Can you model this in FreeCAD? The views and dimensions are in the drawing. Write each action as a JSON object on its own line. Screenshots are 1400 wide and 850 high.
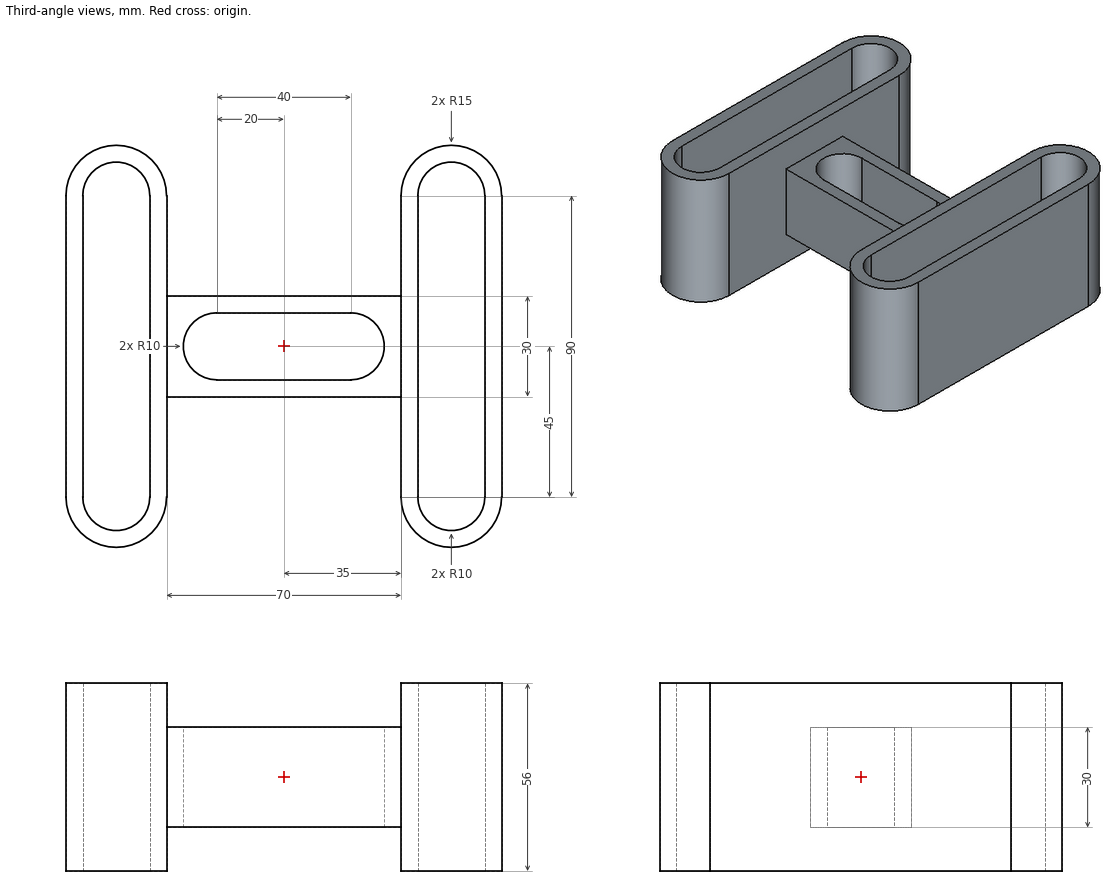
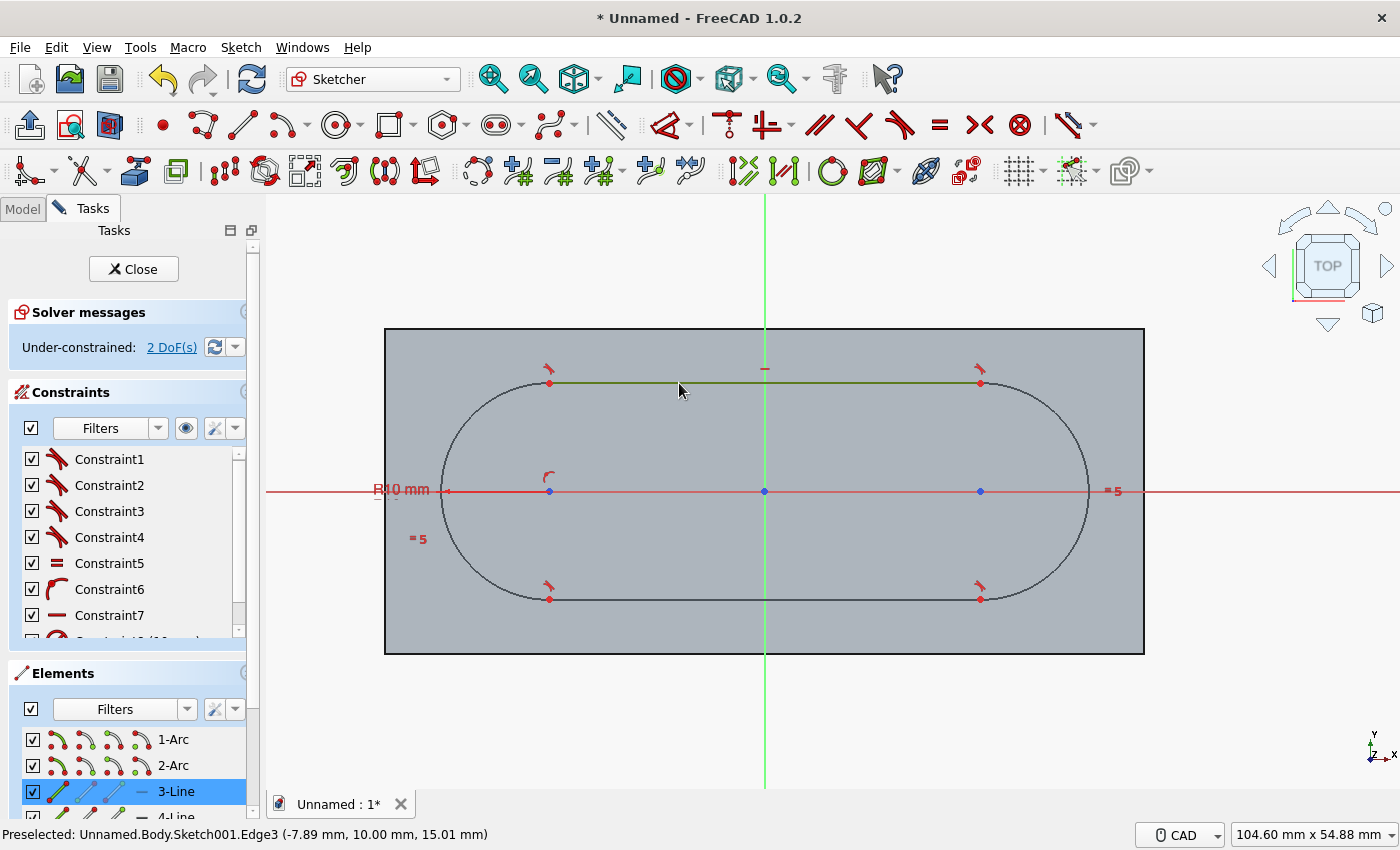
{"action": "key", "text": "l"}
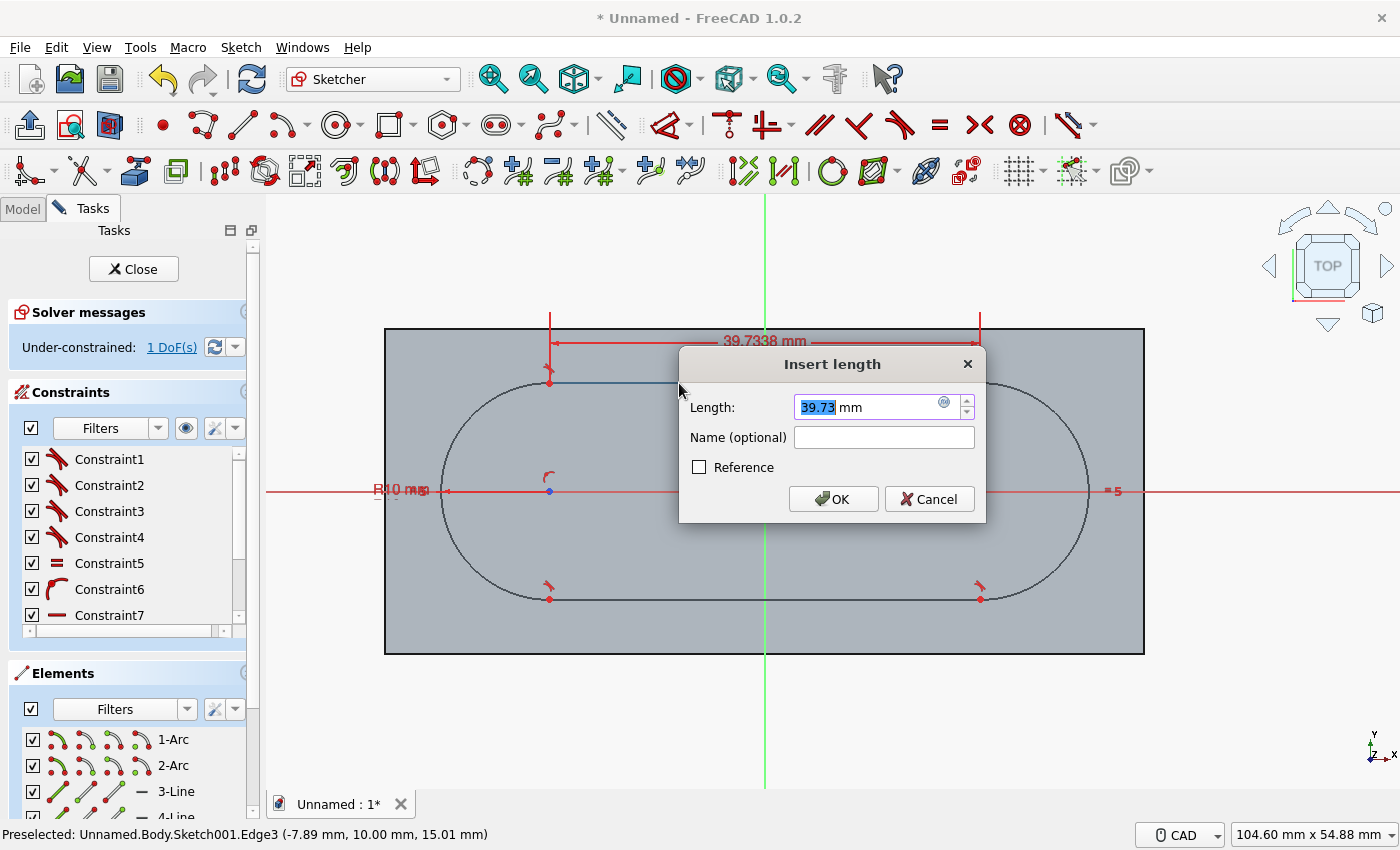
{"action": "type", "text": "40"}
{"action": "key", "text": "Return"}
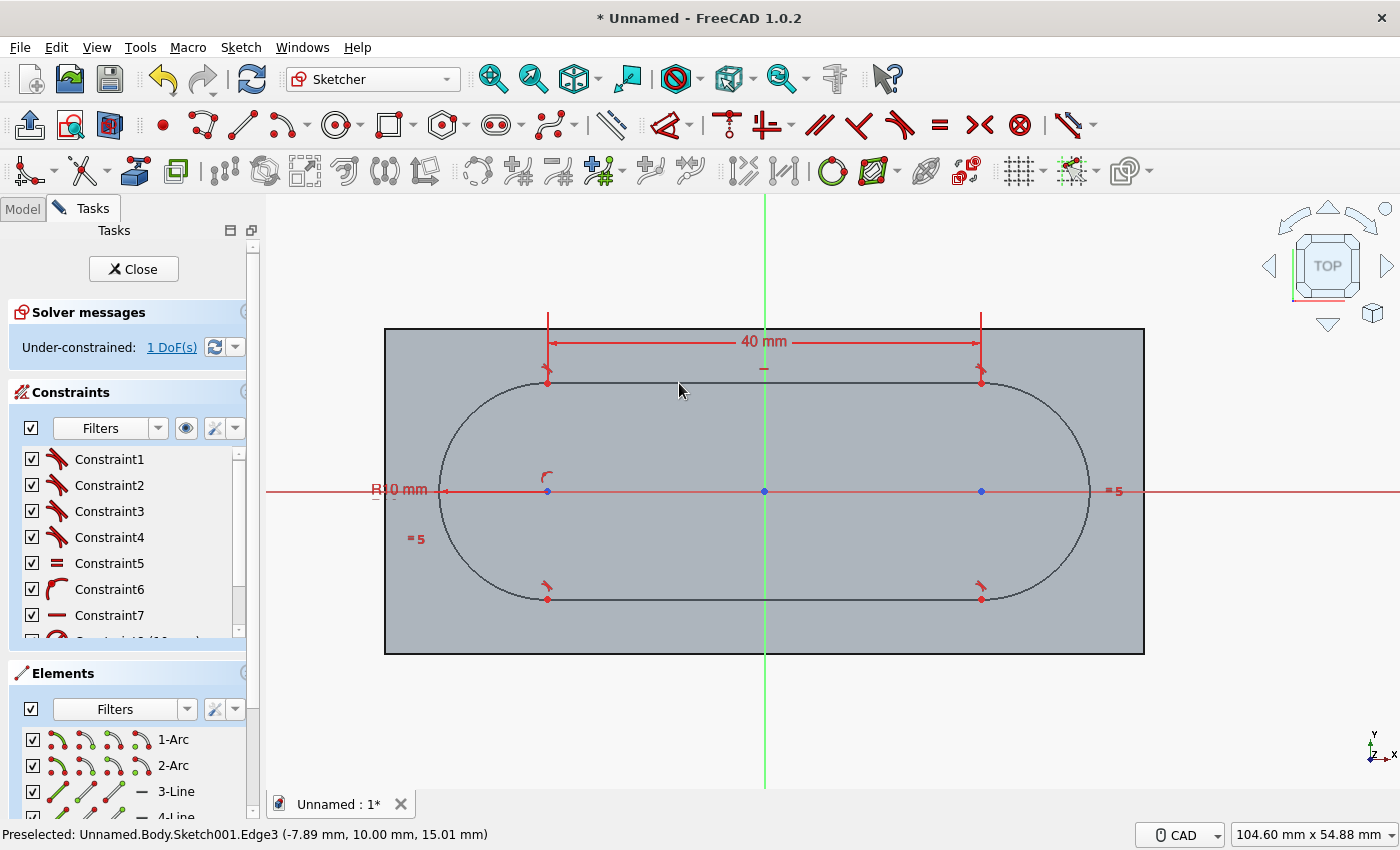
{"action": "left_click", "coordinate": [548, 383]}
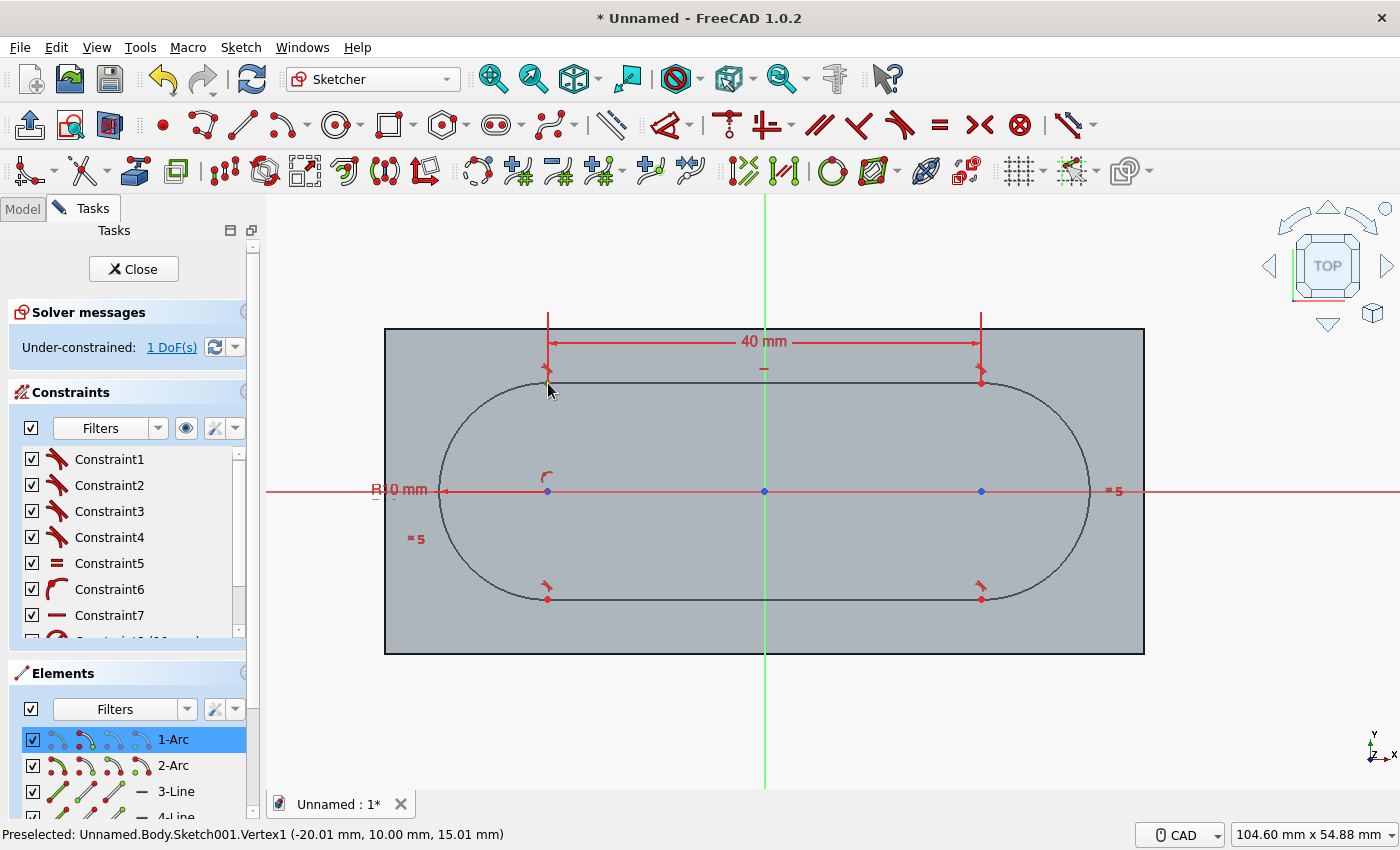
{"action": "key", "text": "l"}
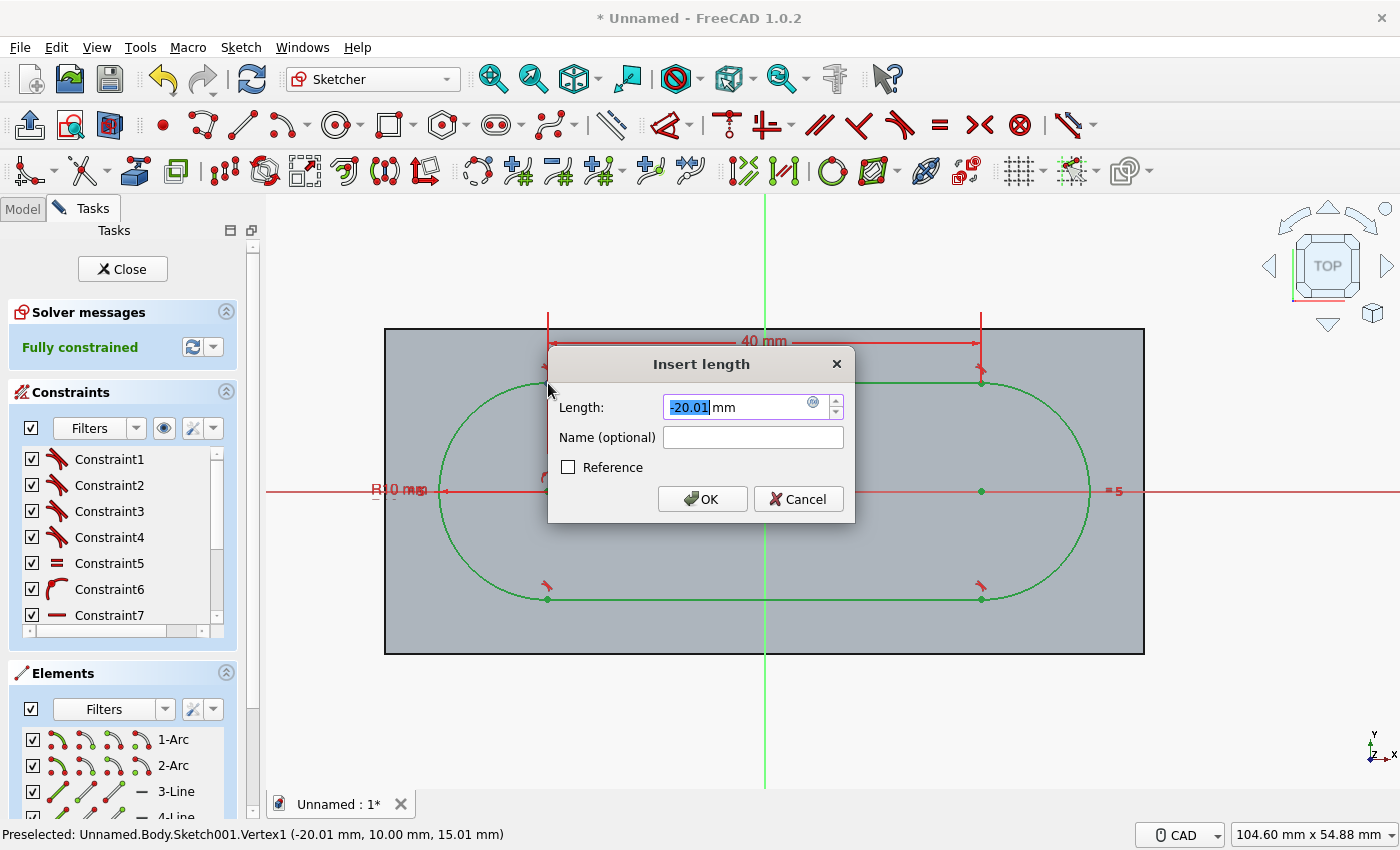
{"action": "type", "text": "-20"}
{"action": "key", "text": "Return"}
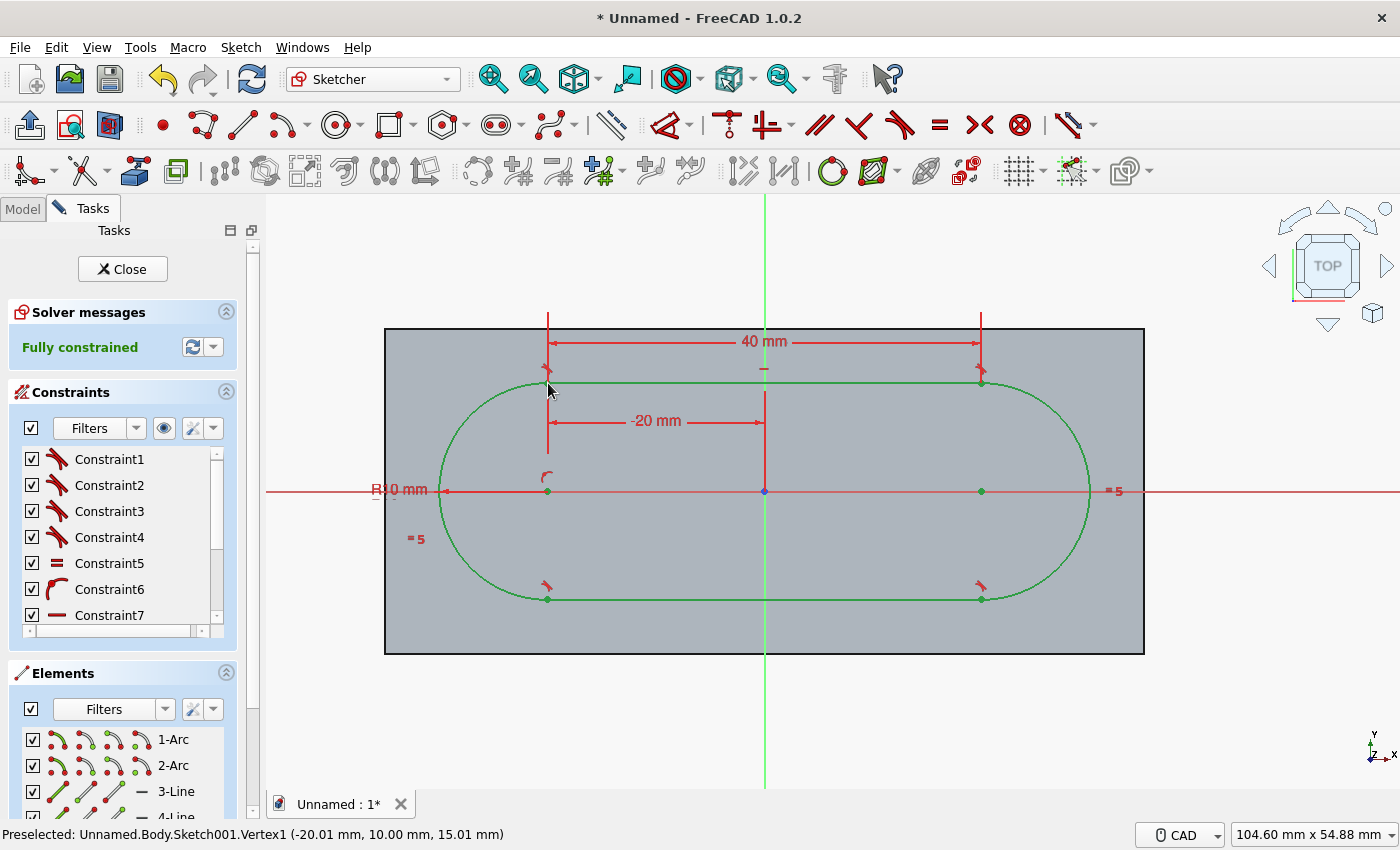
{"action": "left_click", "coordinate": [123, 269]}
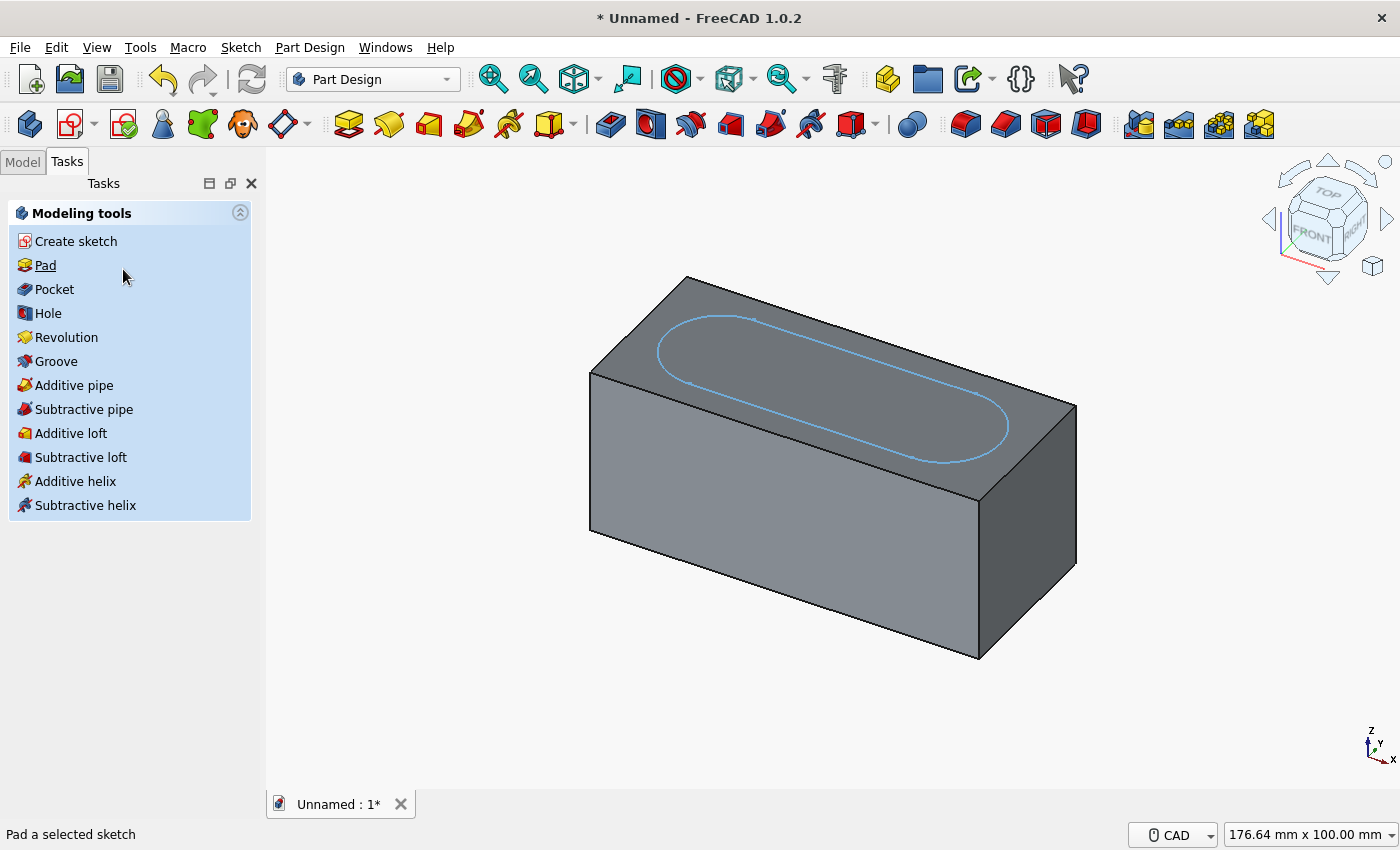
{"action": "left_click", "coordinate": [612, 124]}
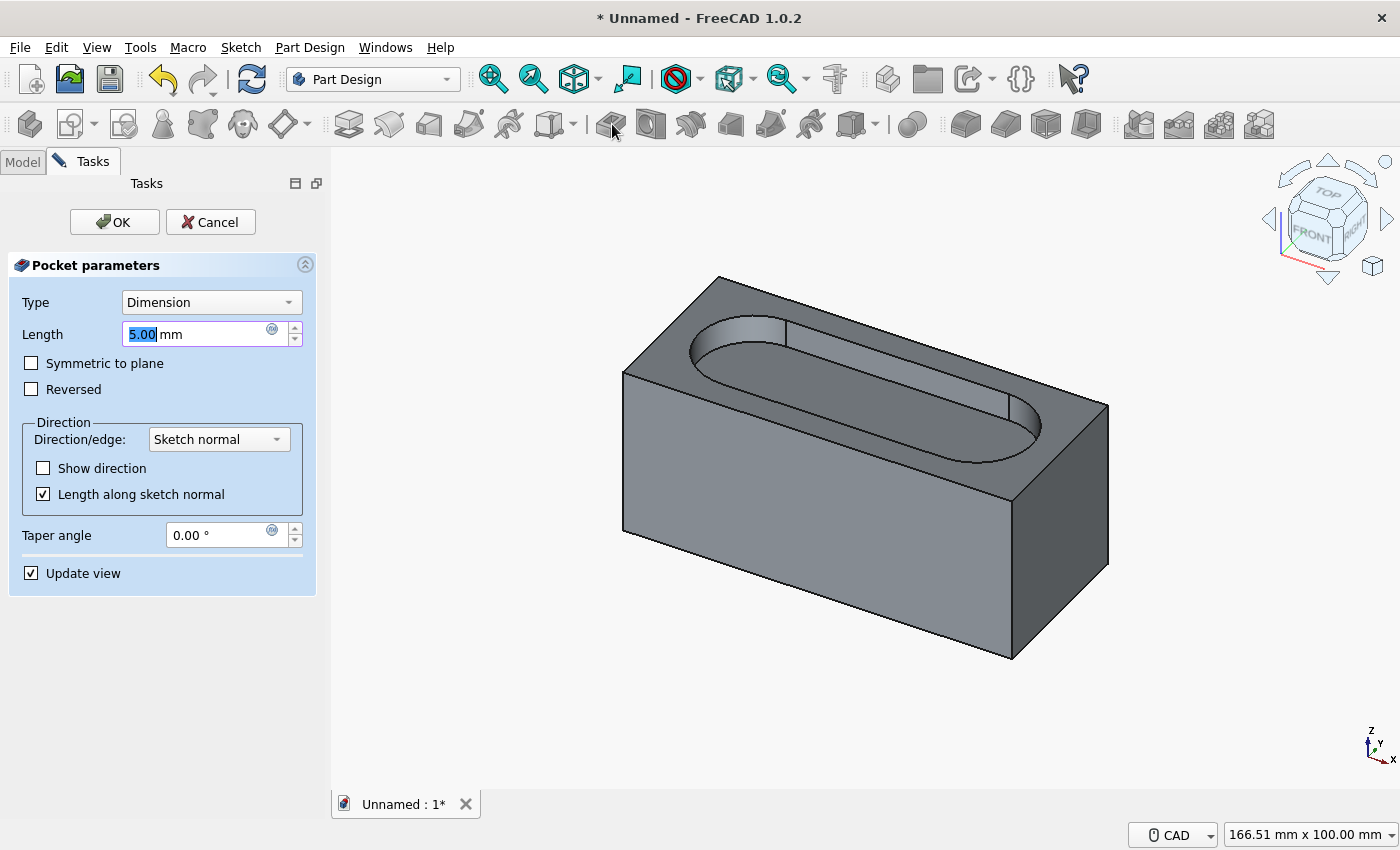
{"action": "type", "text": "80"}
{"action": "key", "text": "Tab"}